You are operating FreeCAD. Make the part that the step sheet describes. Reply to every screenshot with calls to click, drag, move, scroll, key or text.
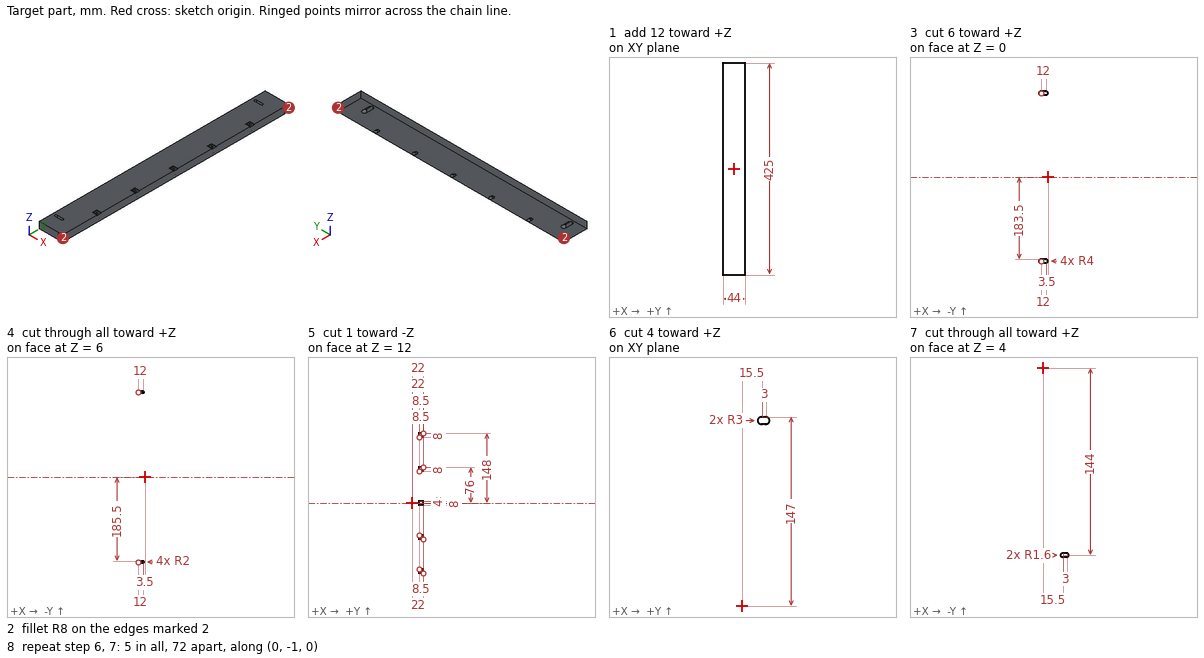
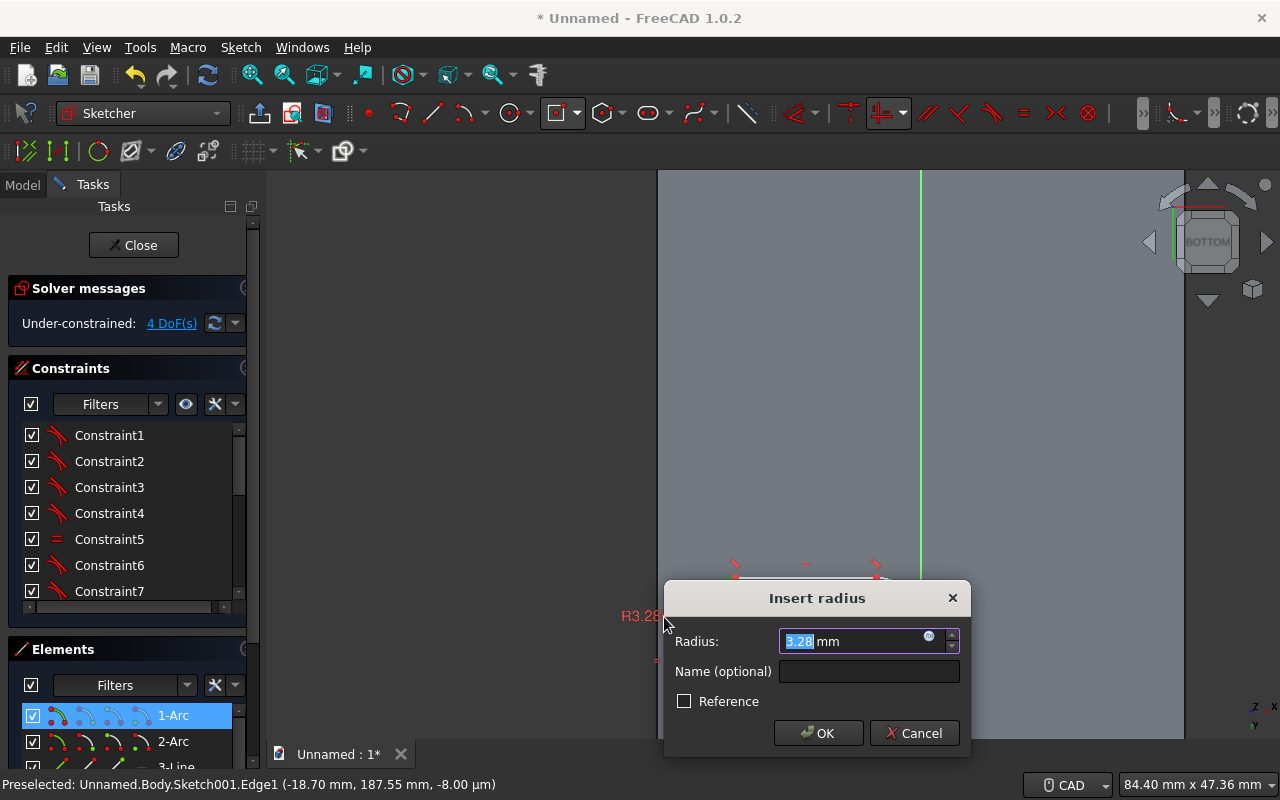
text(4)
key(Return)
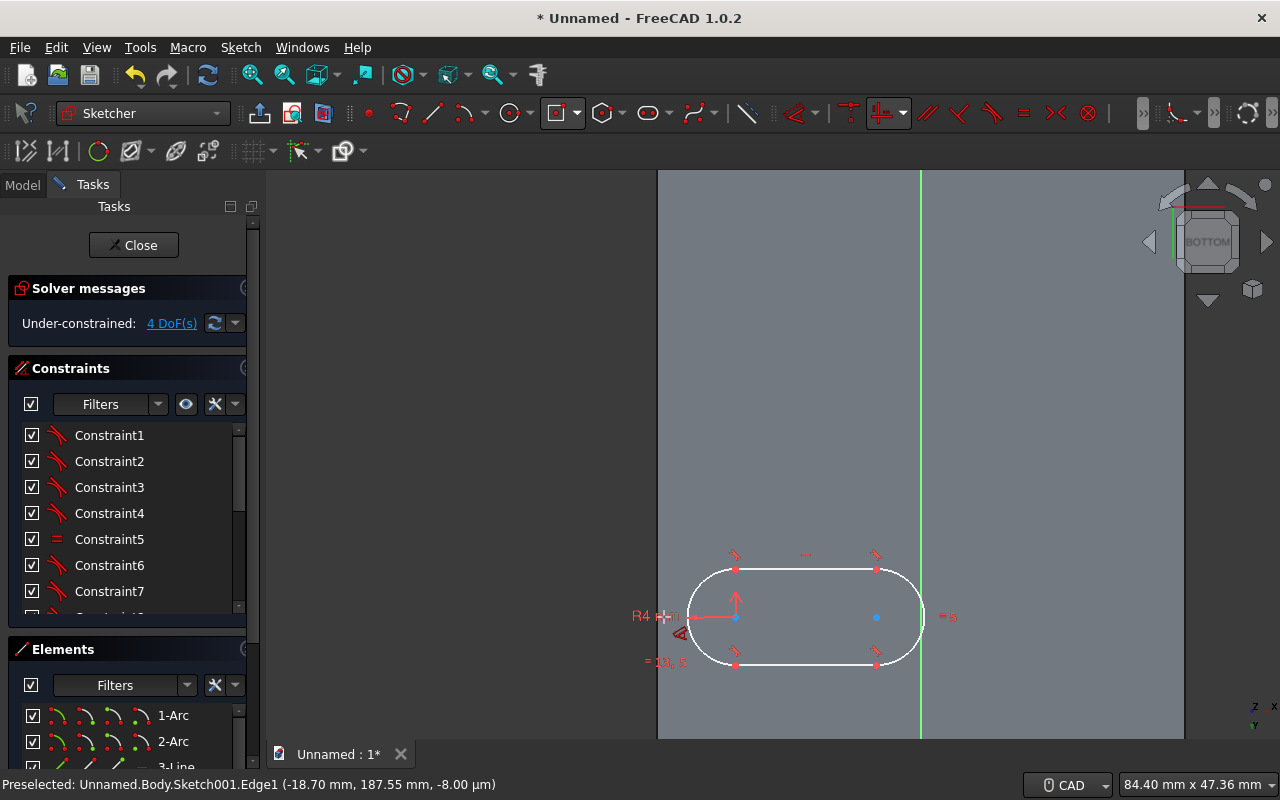
scroll(696, 622, down, 13)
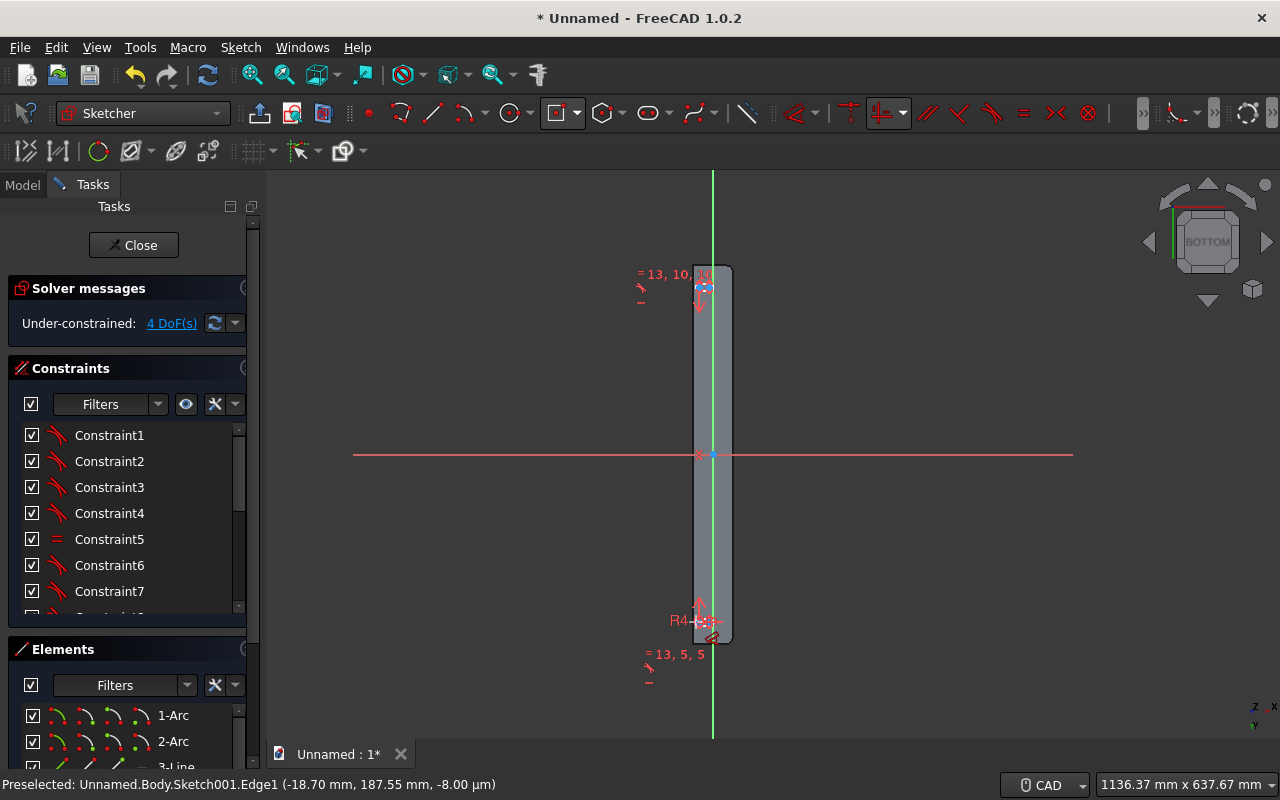
scroll(702, 619, up, 8)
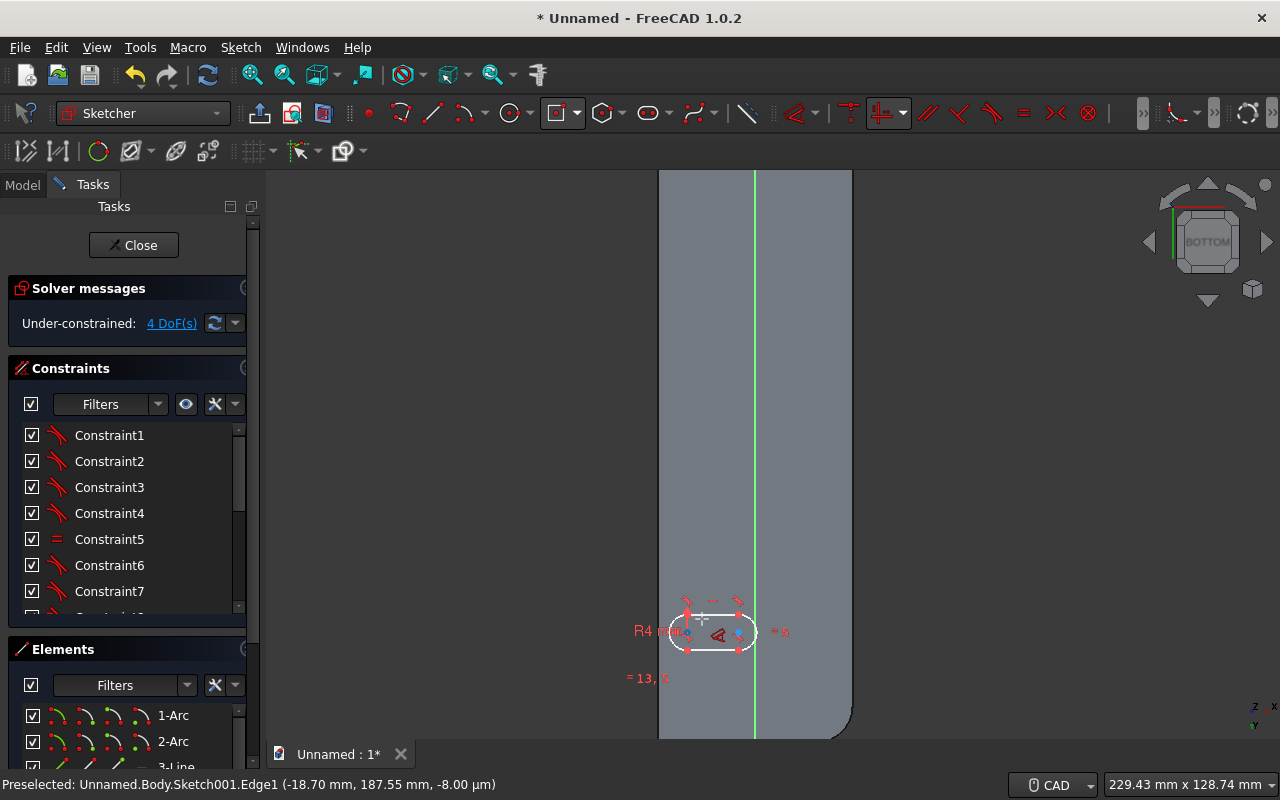
click(703, 615)
click(713, 581)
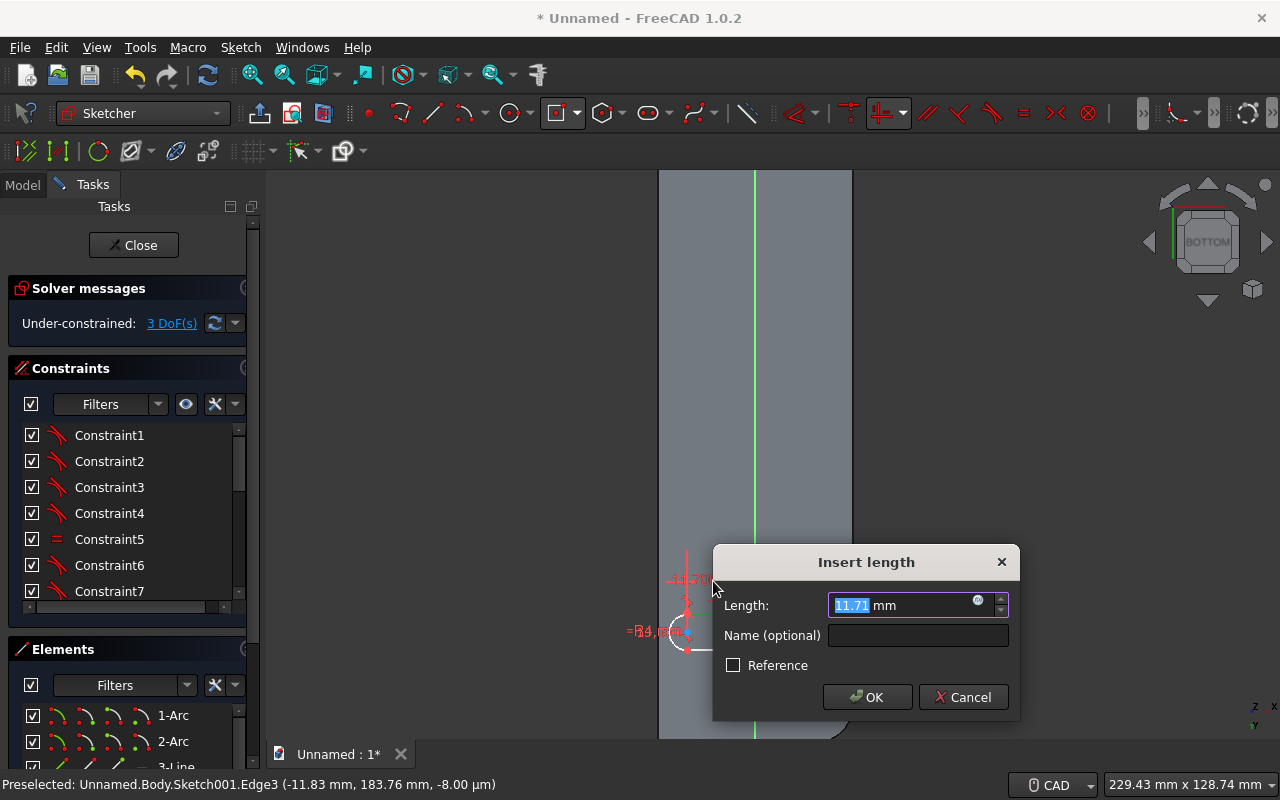
text(12)
key(Return)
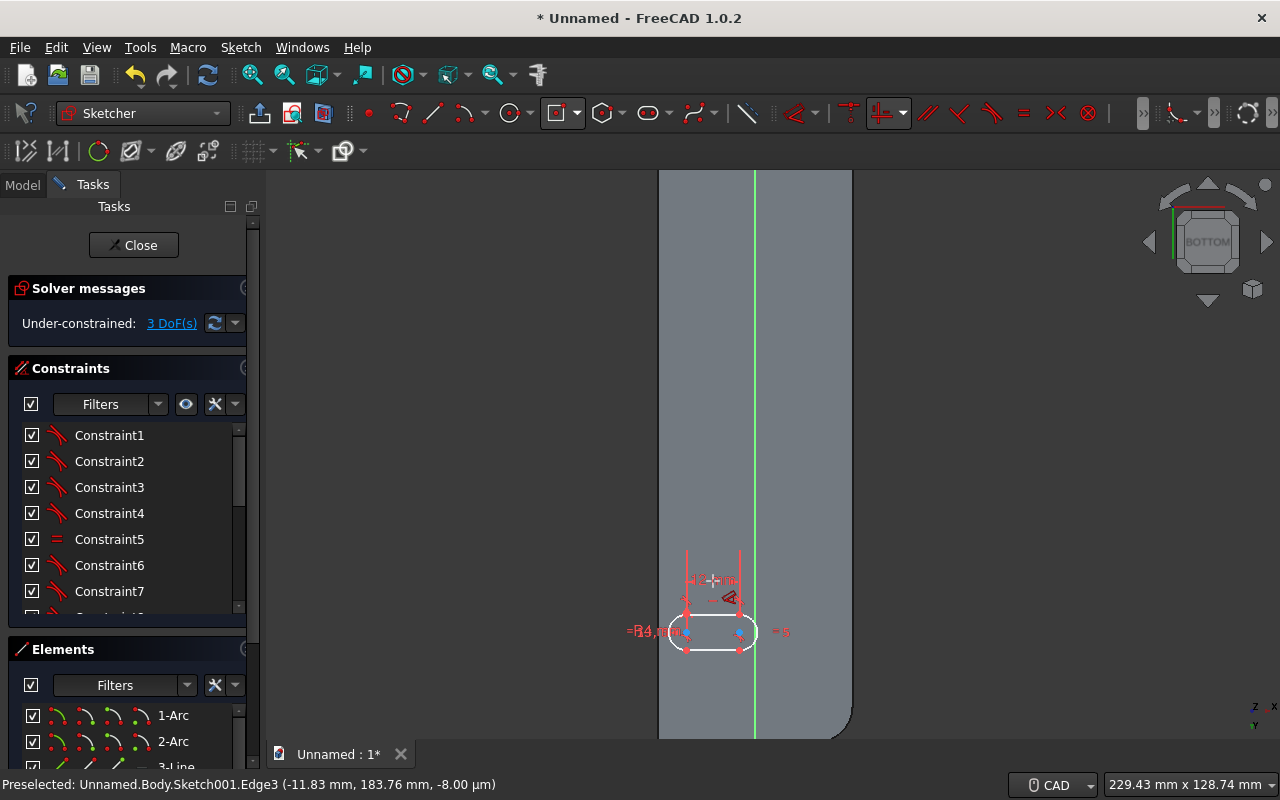
scroll(702, 619, down, 8)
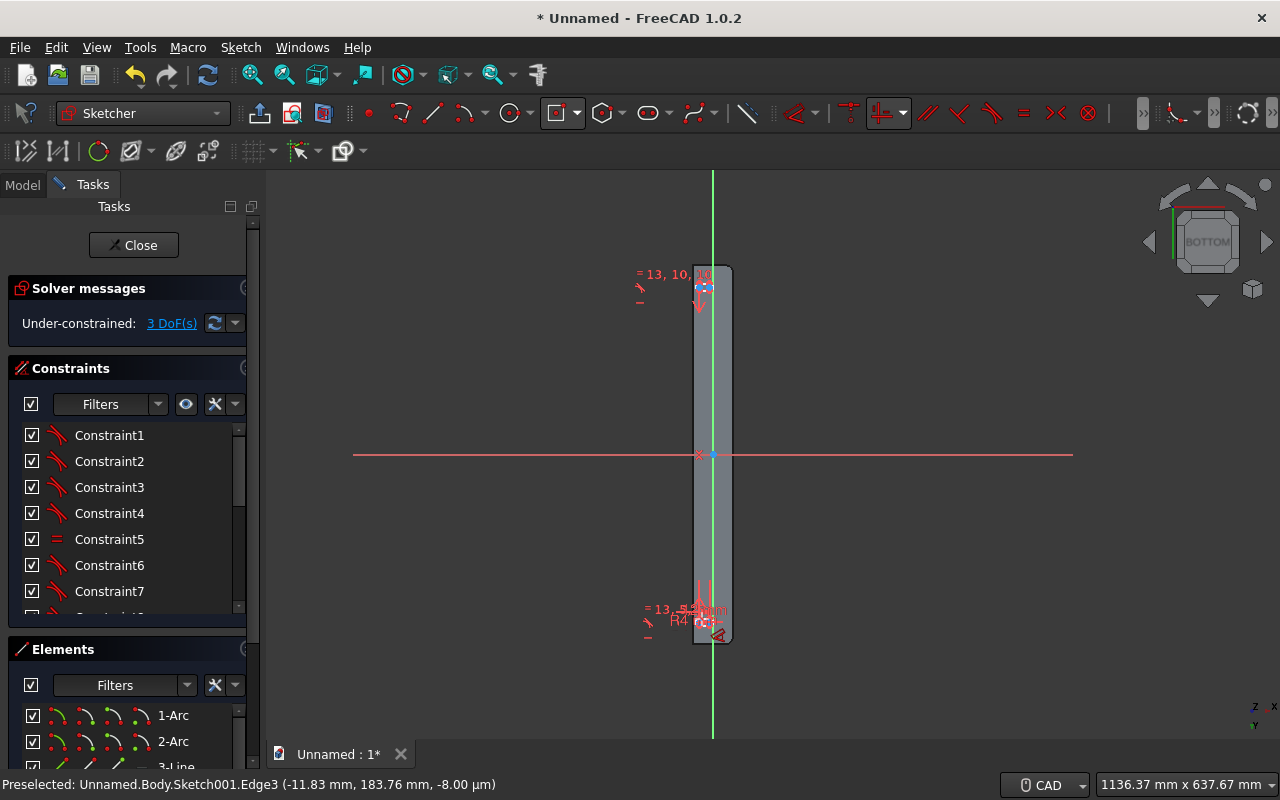
scroll(702, 284, up, 8)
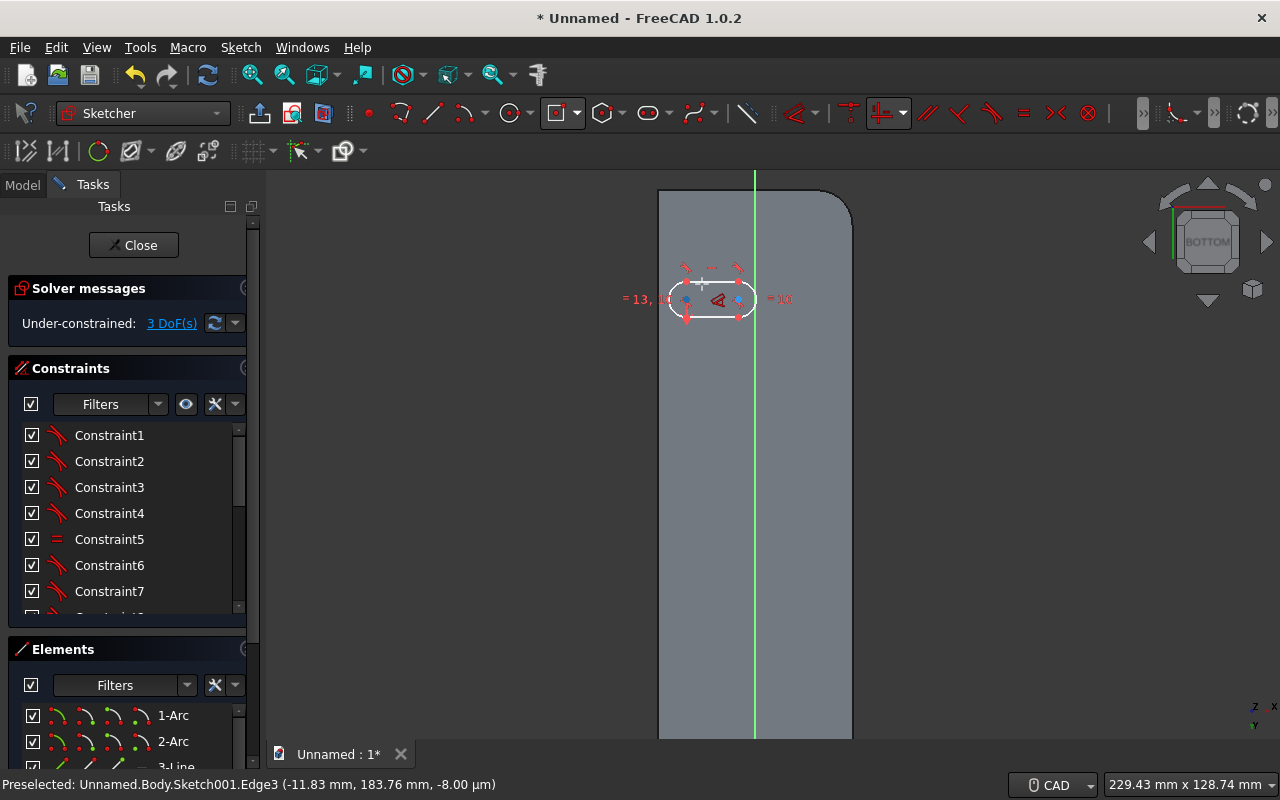
click(702, 282)
click(713, 248)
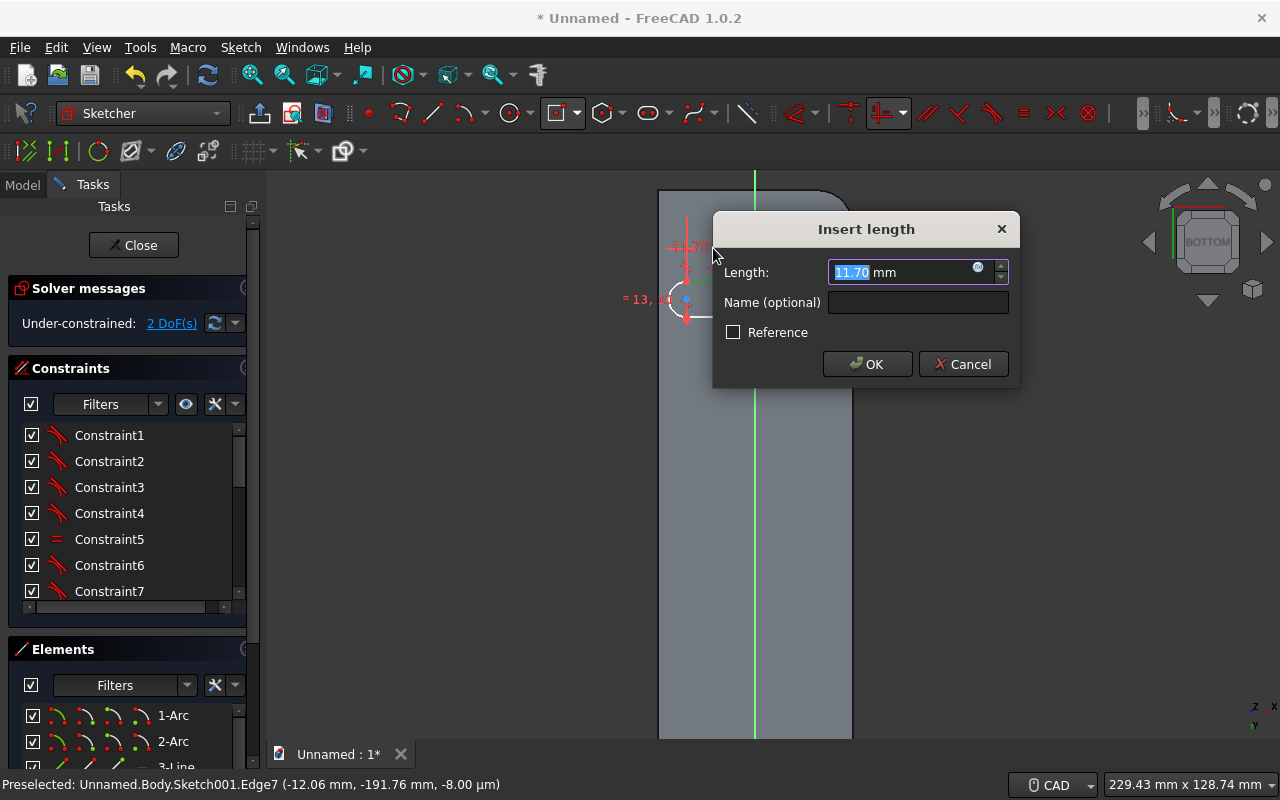
text(12)
key(Return)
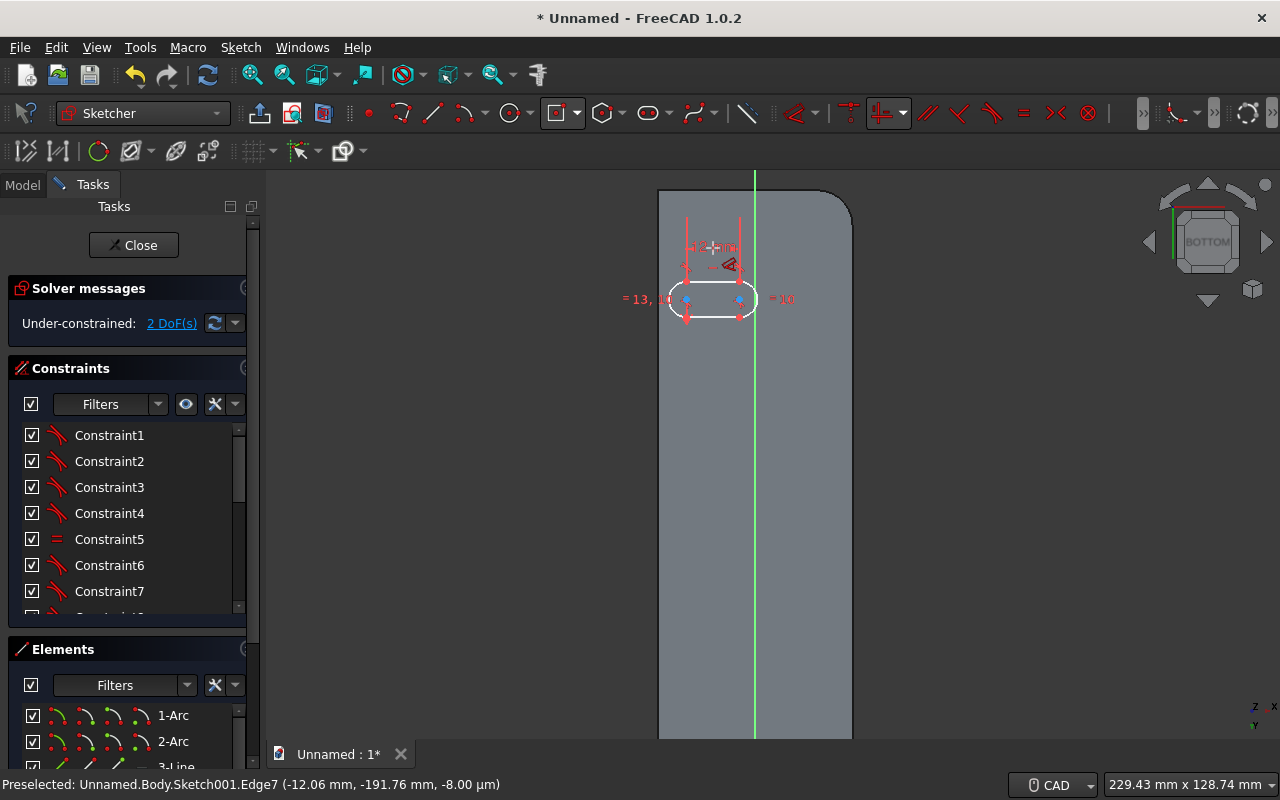
scroll(702, 284, down, 8)